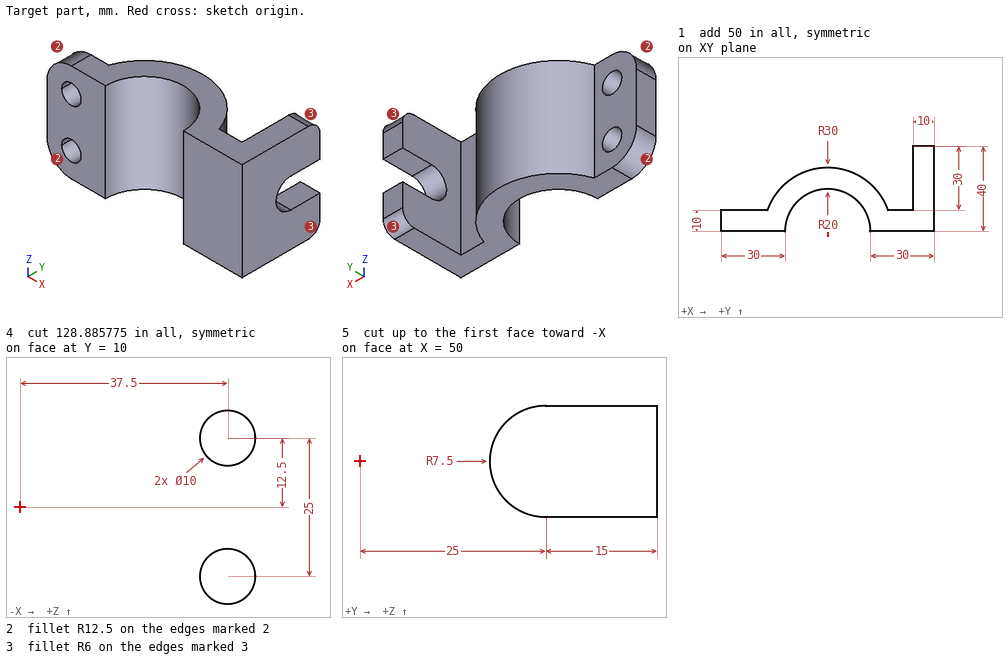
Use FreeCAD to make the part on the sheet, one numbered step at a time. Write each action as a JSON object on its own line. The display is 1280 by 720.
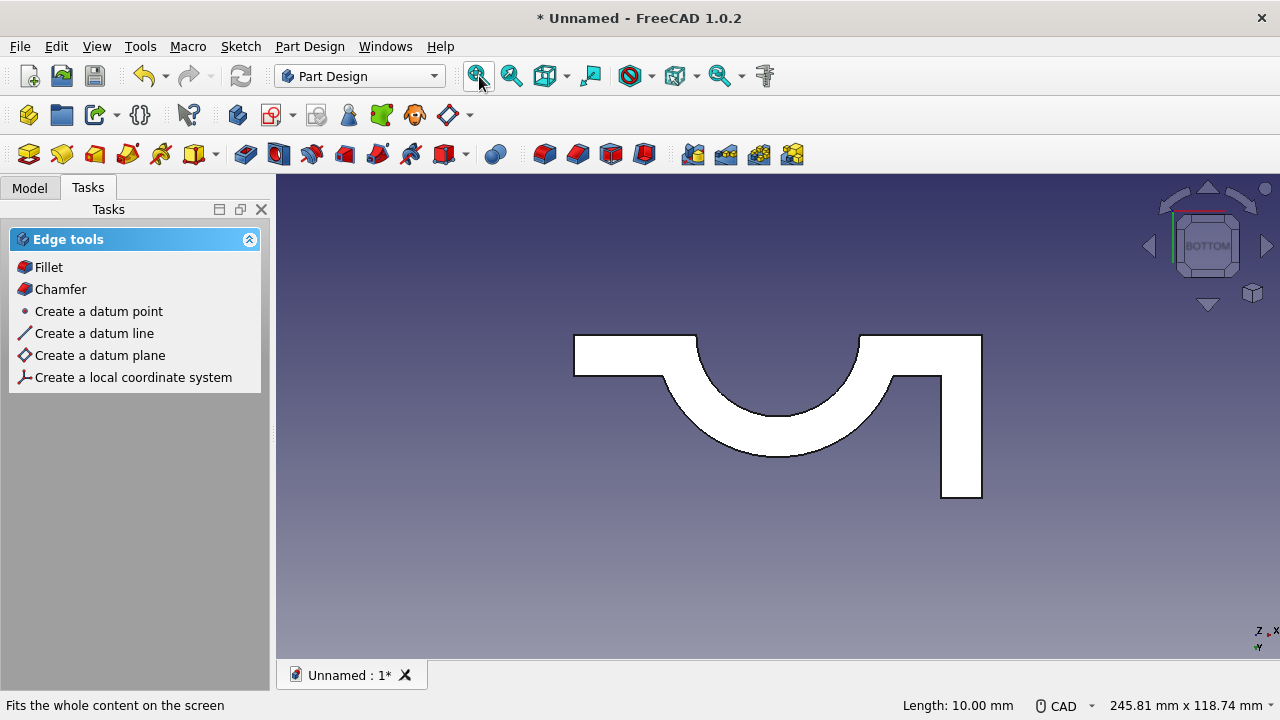
{"action": "left_click", "coordinate": [574, 354], "text": "ctrl"}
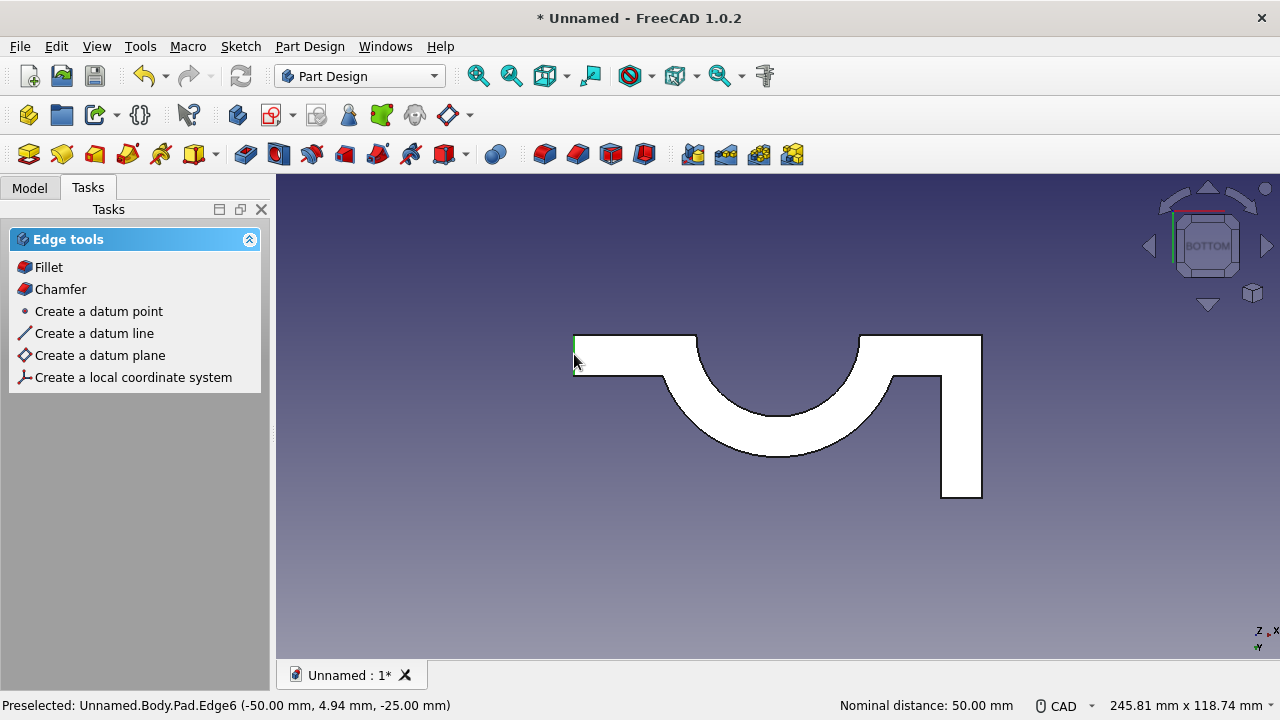
{"action": "left_click", "coordinate": [545, 154]}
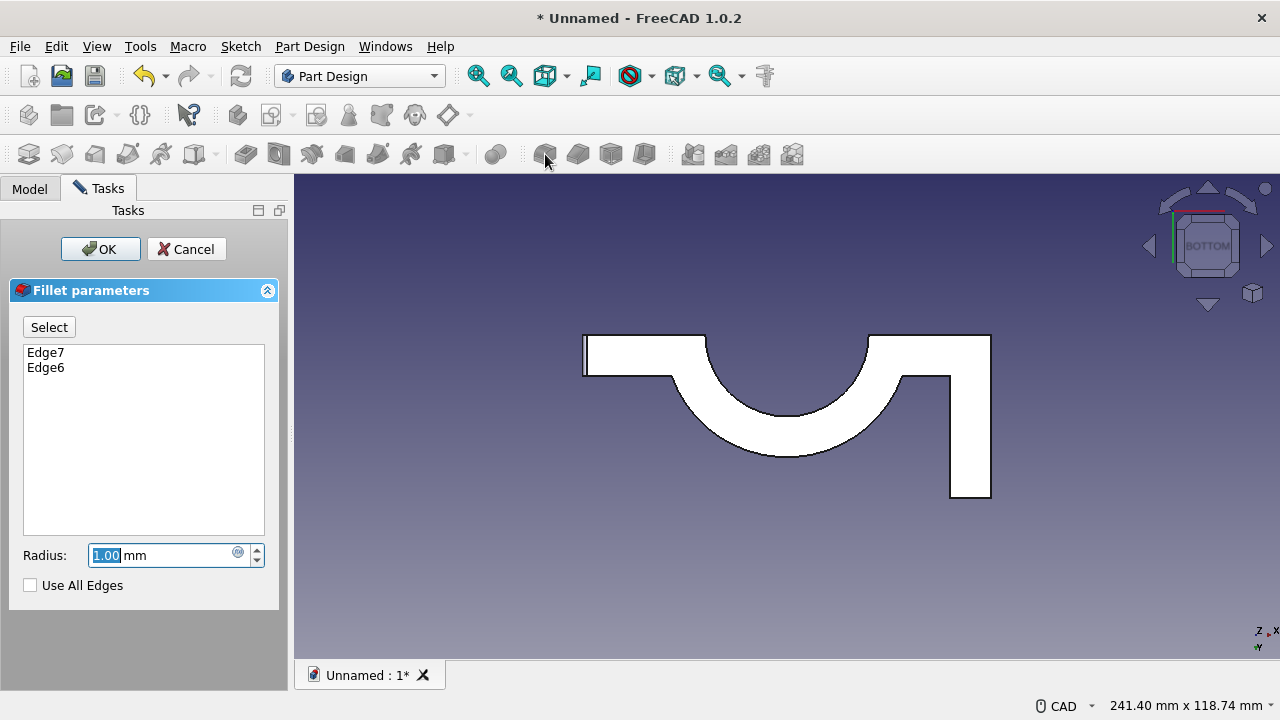
{"action": "type", "text": "12.5"}
{"action": "key", "text": "Tab"}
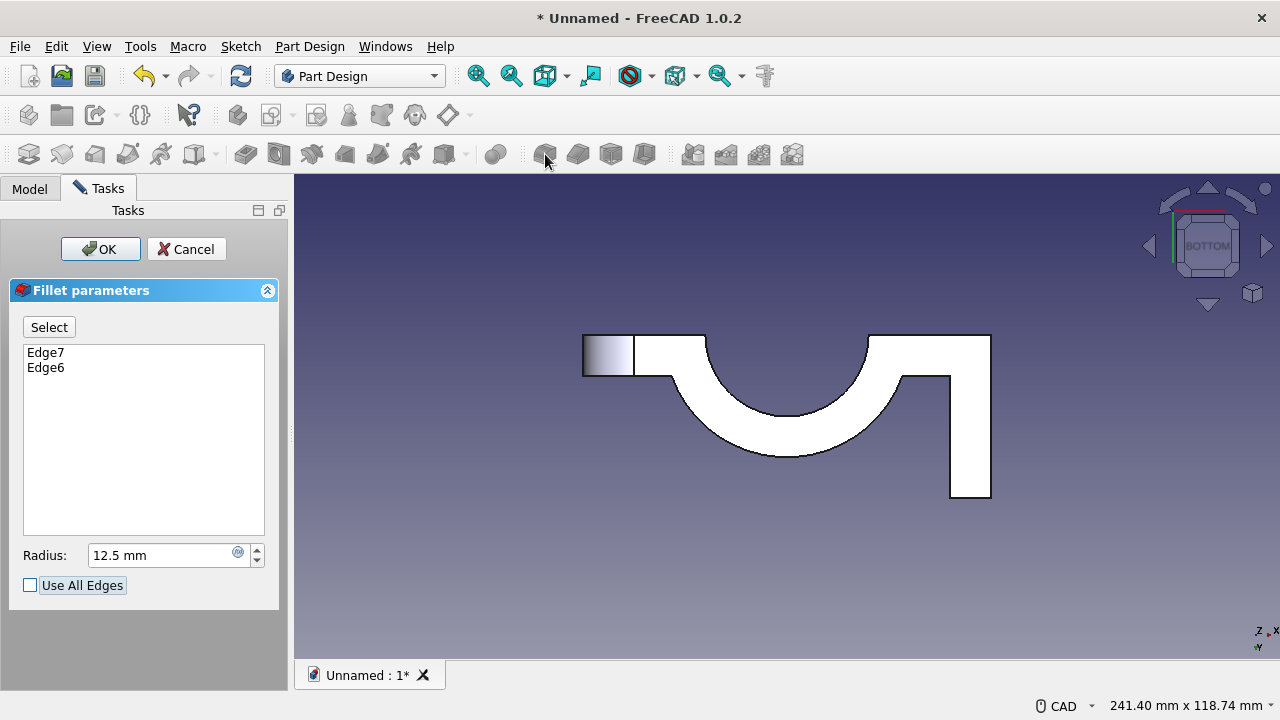
{"action": "left_click", "coordinate": [101, 249]}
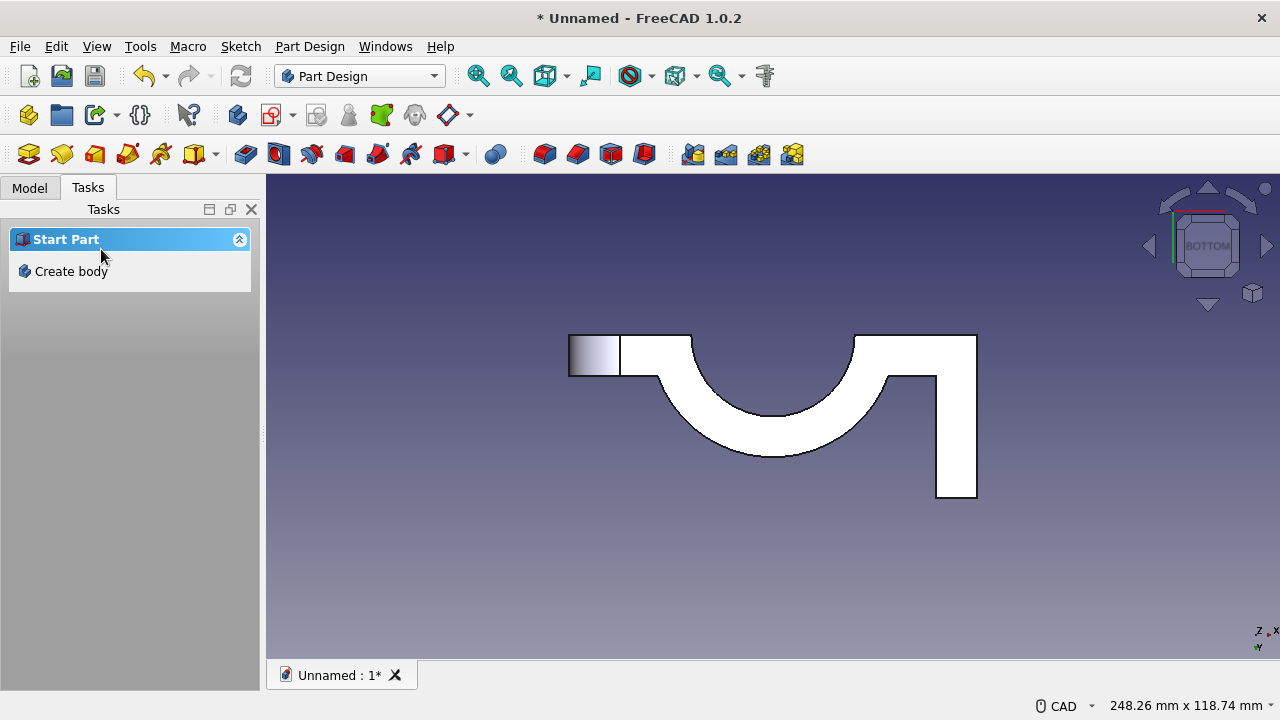
{"action": "left_click", "coordinate": [479, 76]}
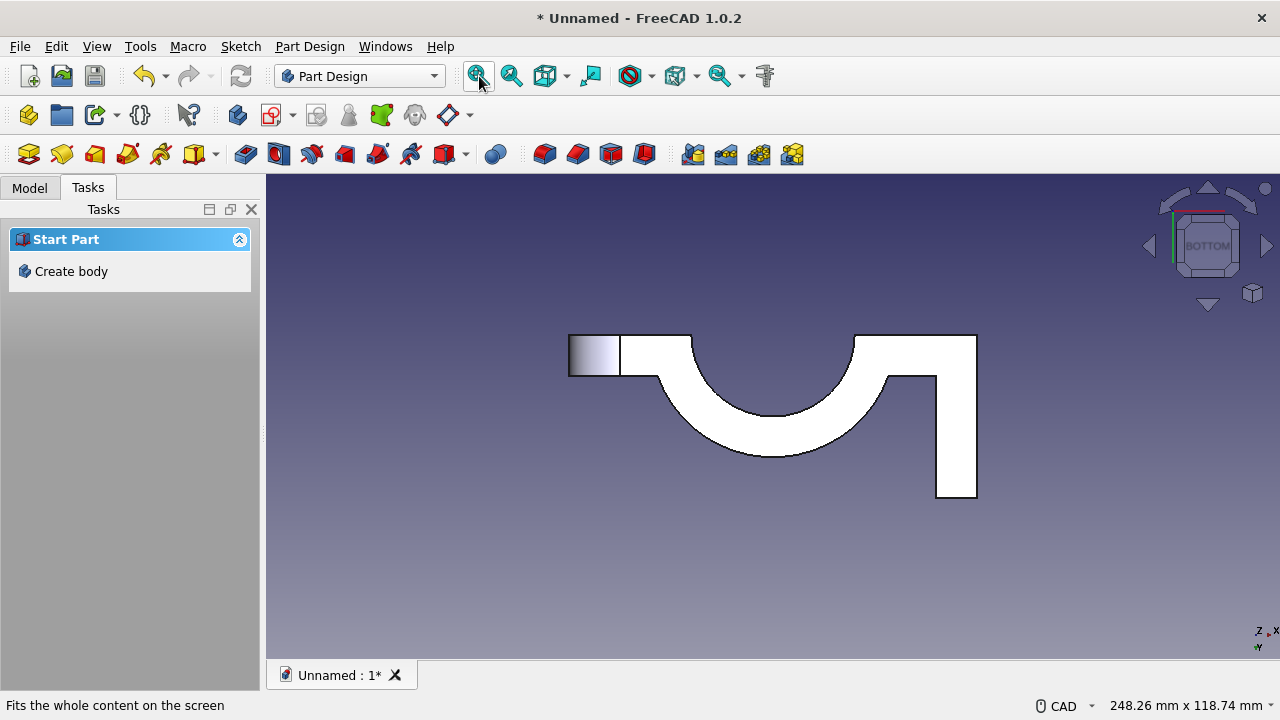
{"action": "left_click", "coordinate": [957, 497]}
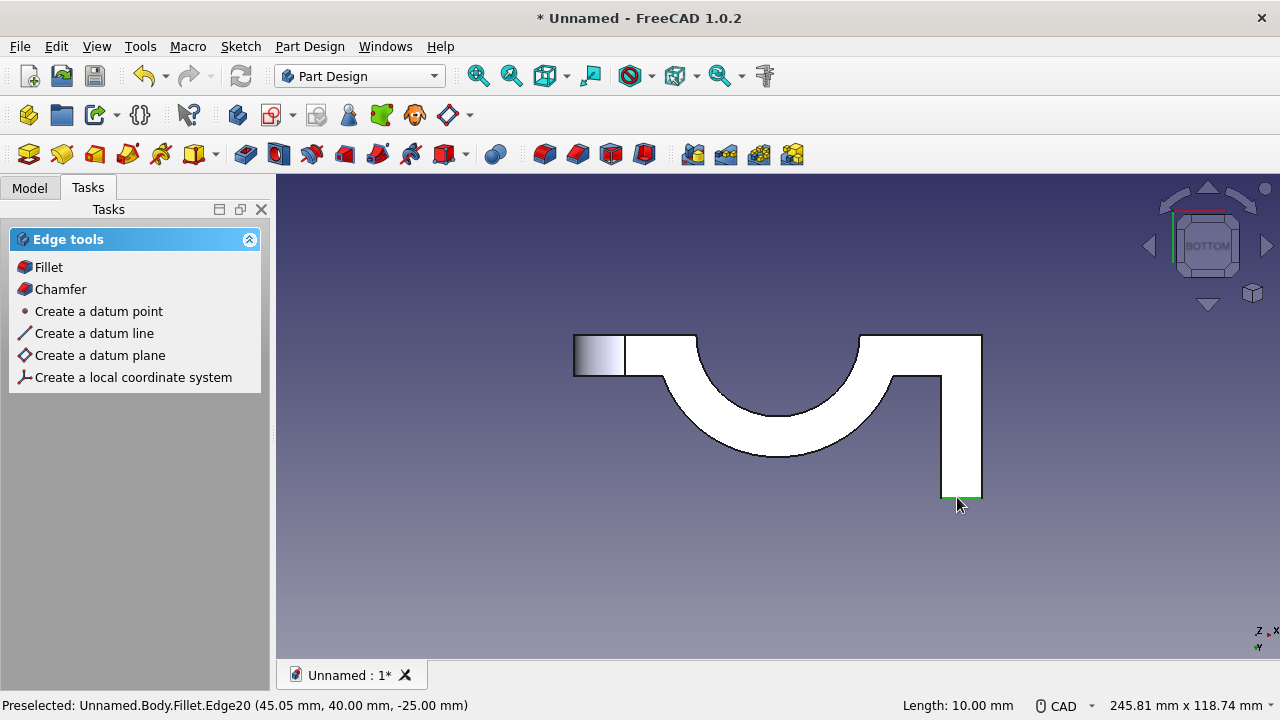
{"action": "key", "text": "0"}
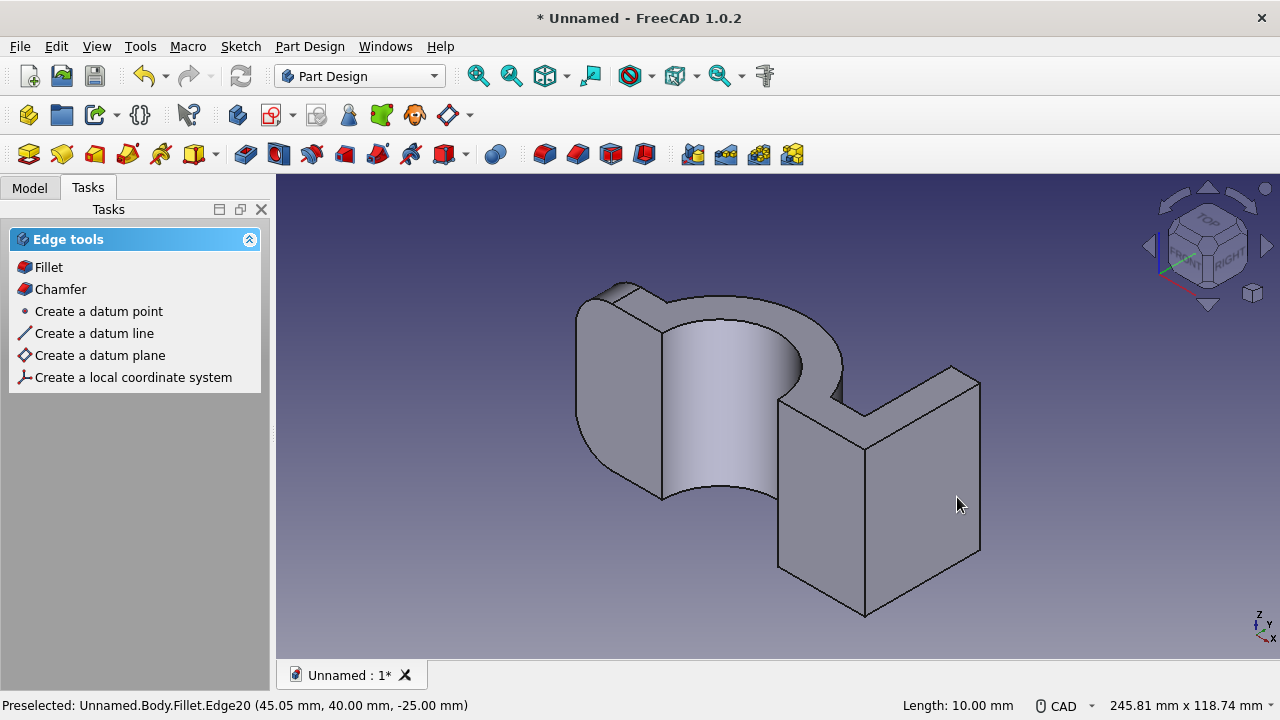
{"action": "key", "text": "2"}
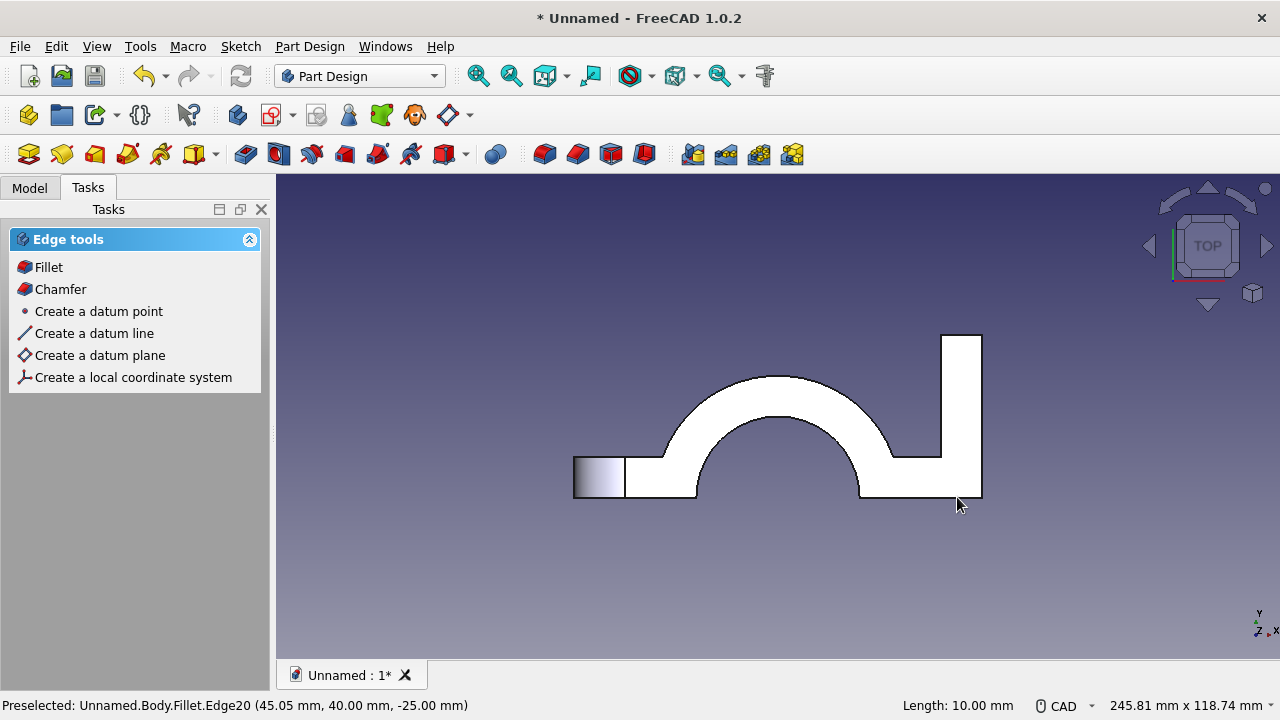
{"action": "left_click", "coordinate": [479, 76]}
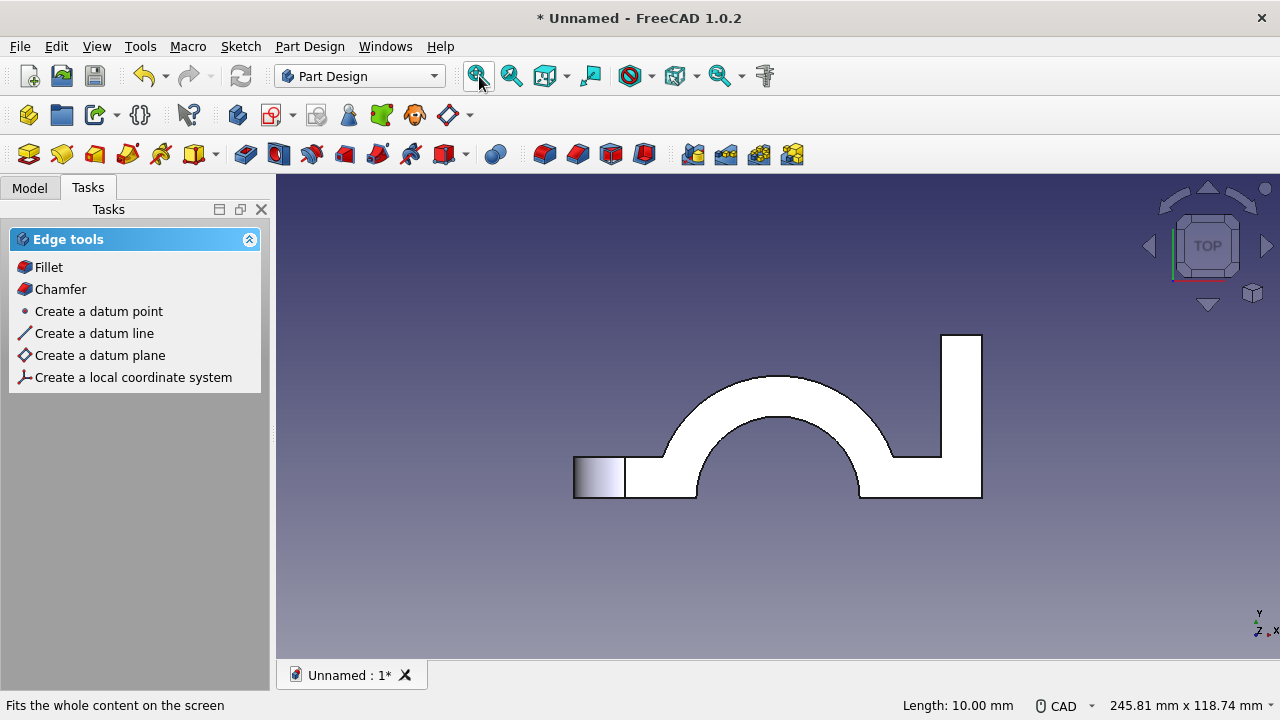
{"action": "left_click", "coordinate": [962, 334], "text": "ctrl"}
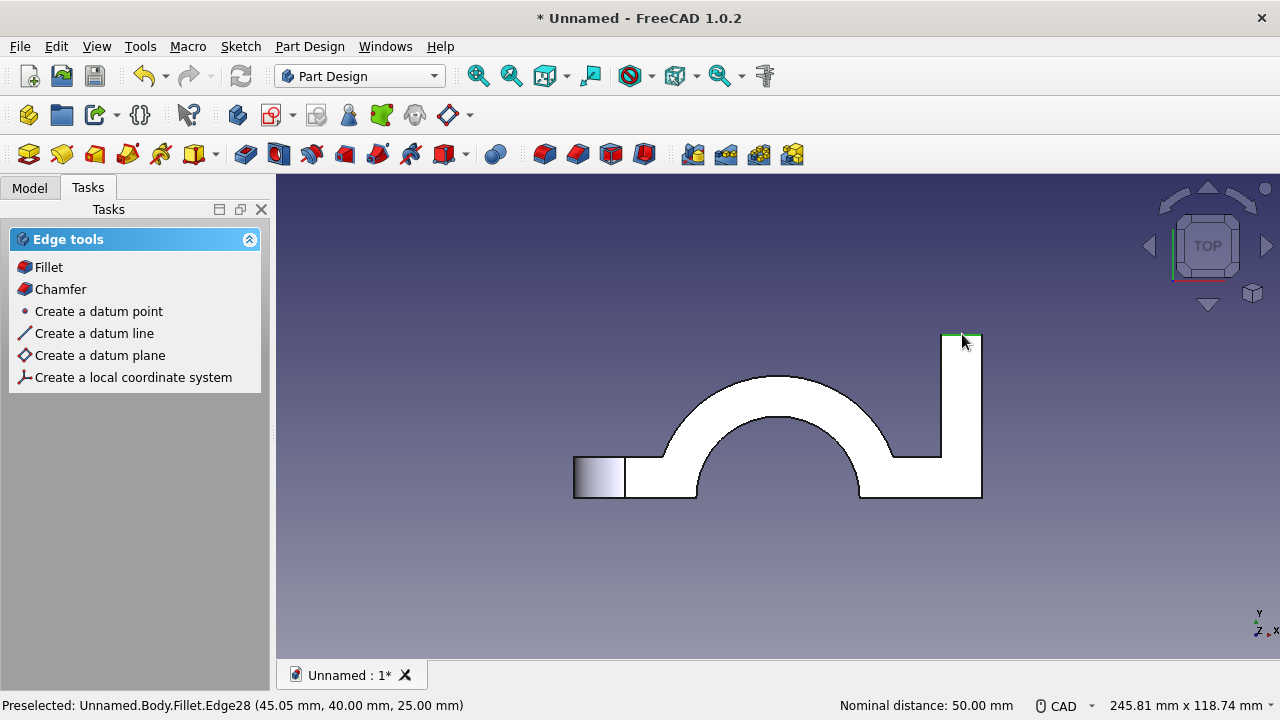
{"action": "left_click", "coordinate": [545, 154]}